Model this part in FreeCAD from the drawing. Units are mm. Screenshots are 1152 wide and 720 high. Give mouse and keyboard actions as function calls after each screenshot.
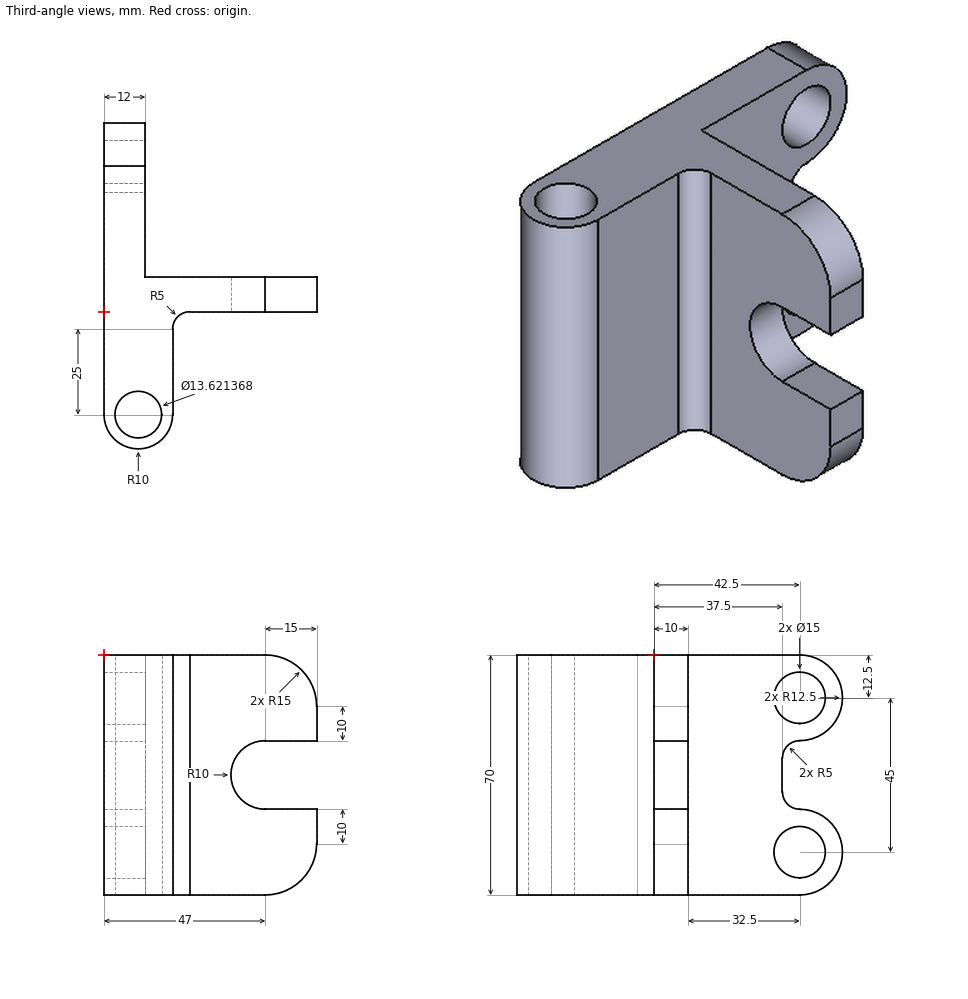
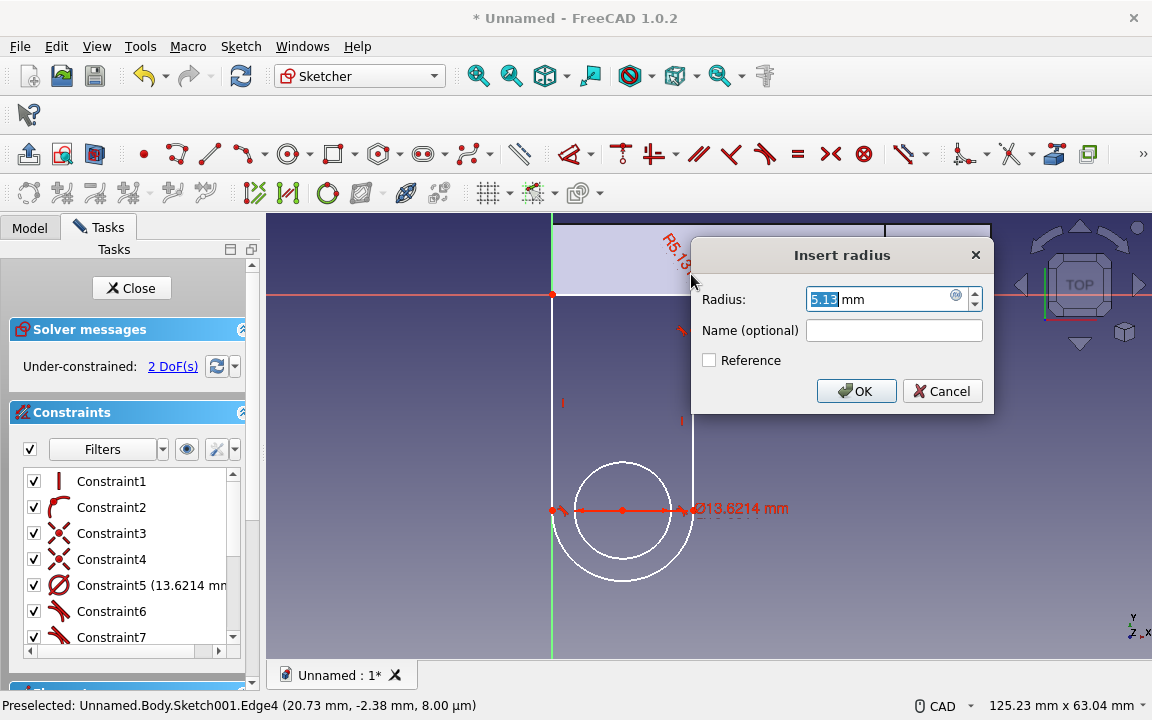
text(5)
key(Return)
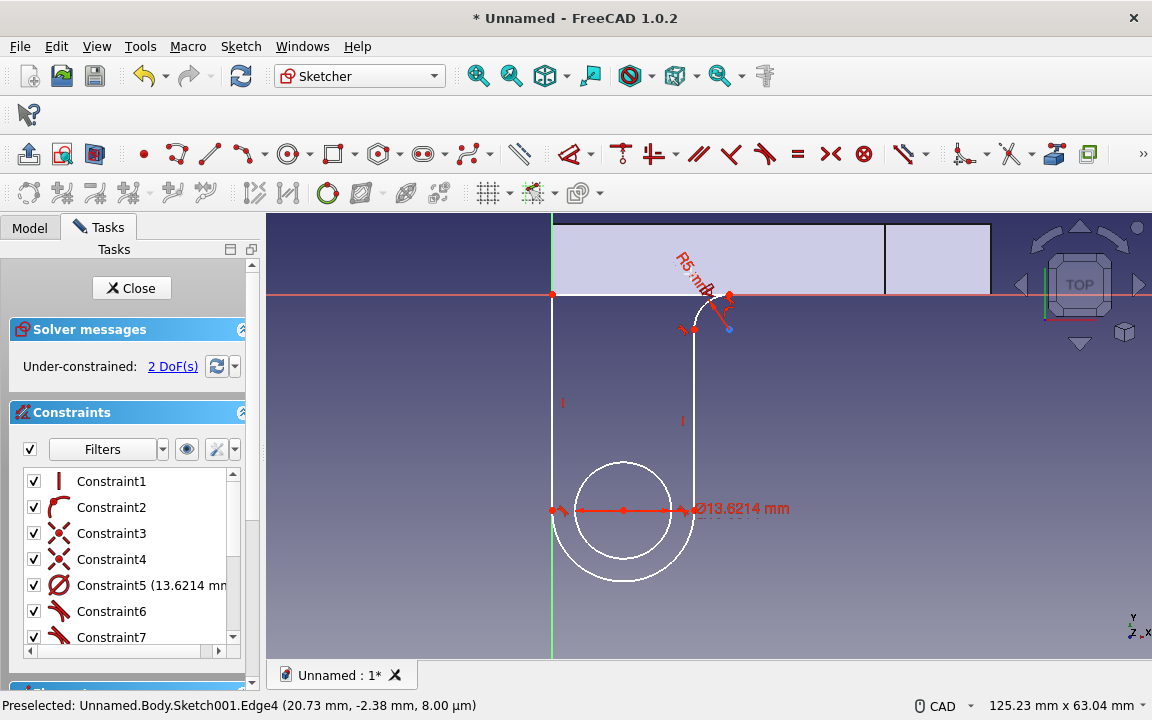
click(582, 568)
click(531, 555)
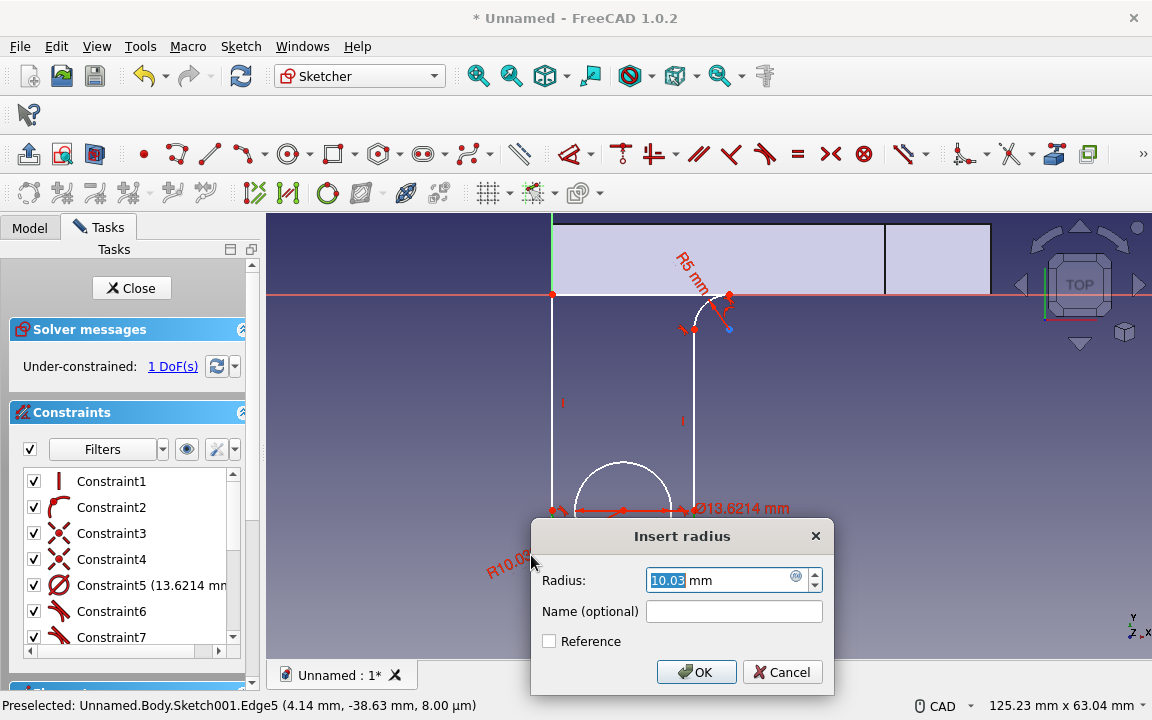
text(10)
key(Return)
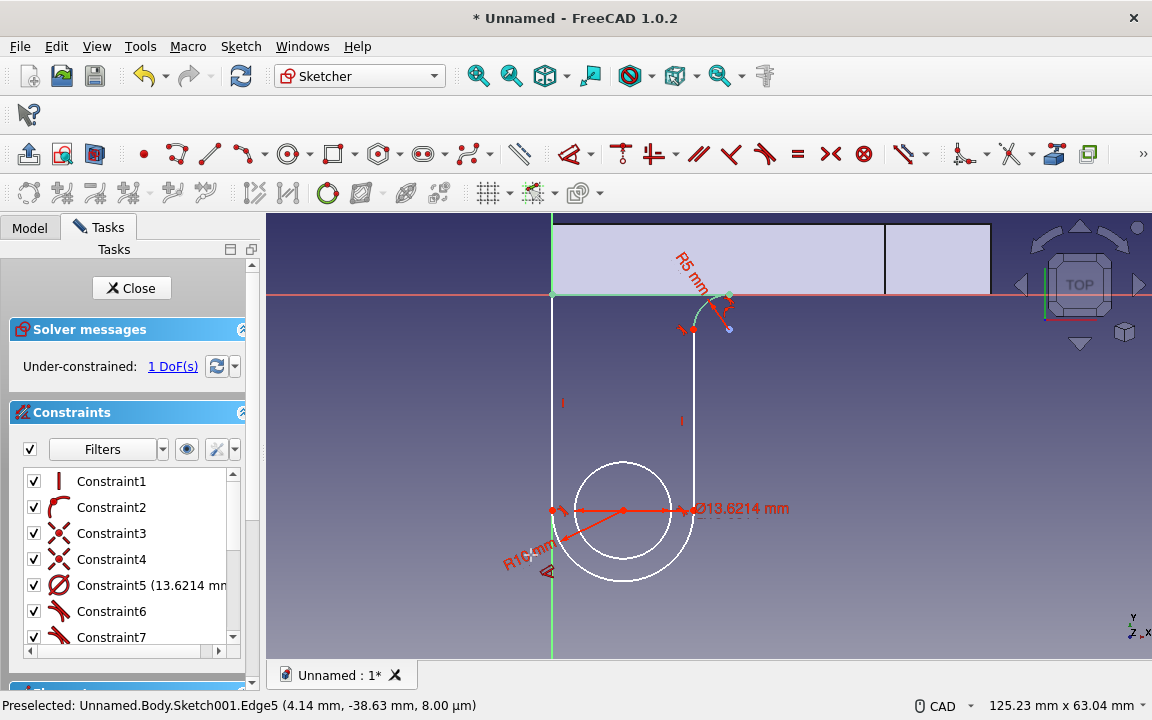
click(694, 456)
click(728, 420)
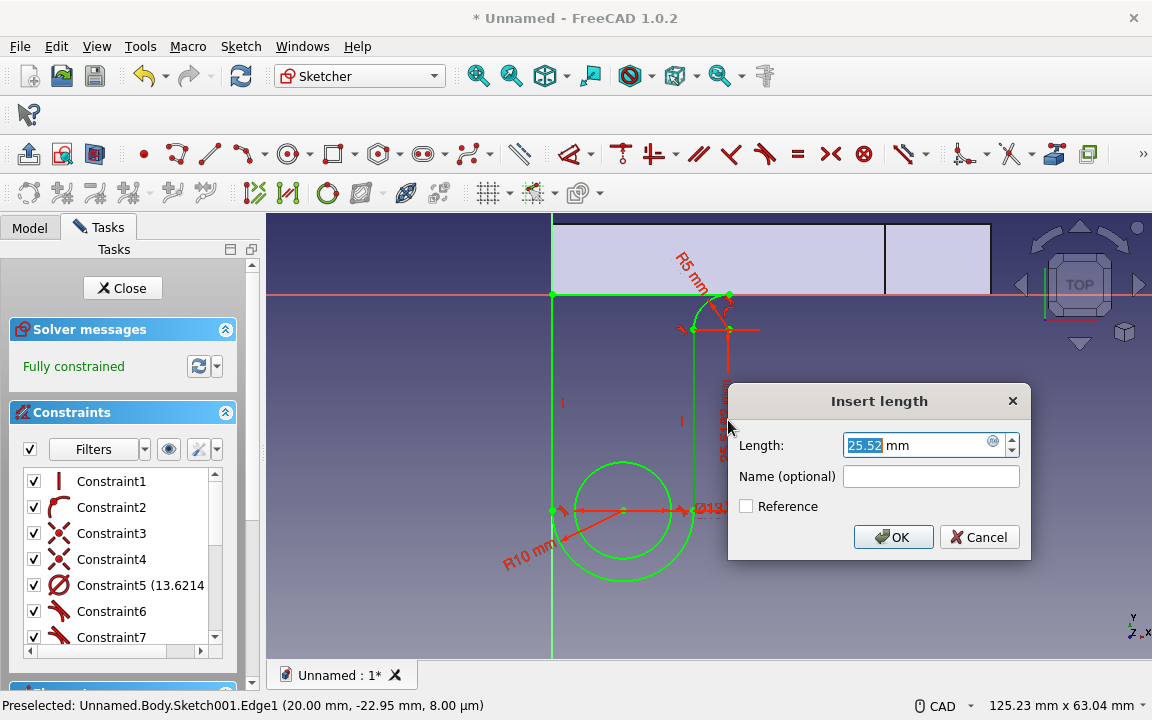
text(25)
key(Return)
key(Escape)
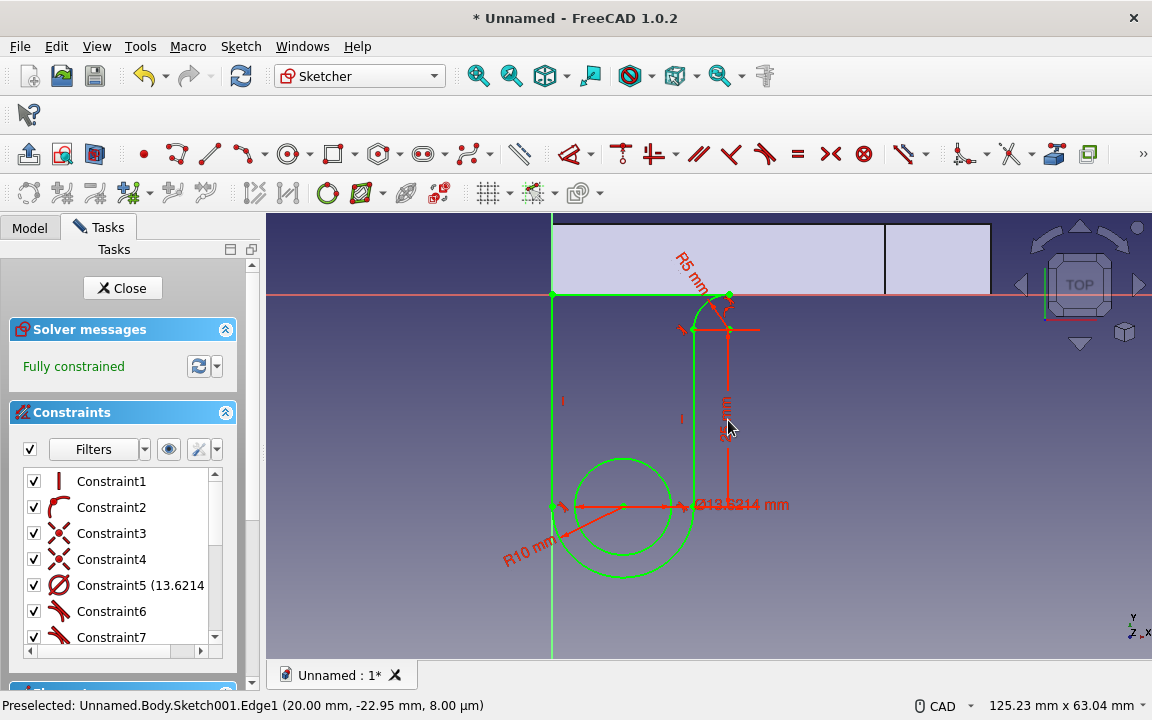
click(123, 288)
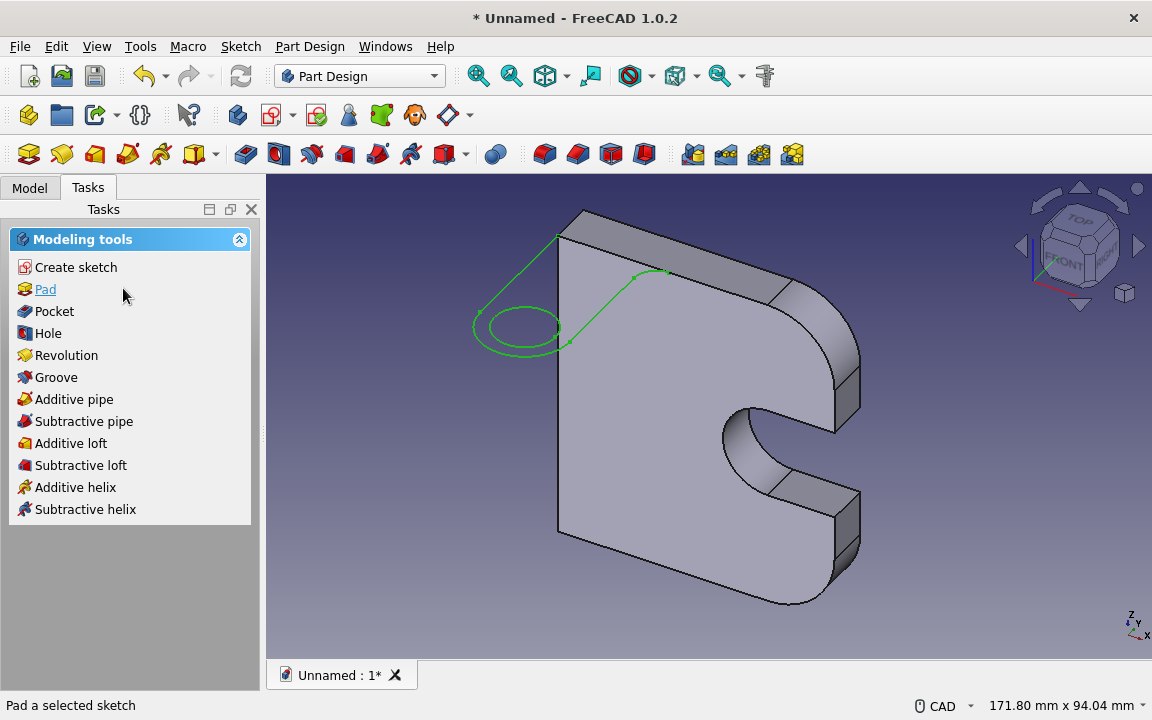
click(29, 154)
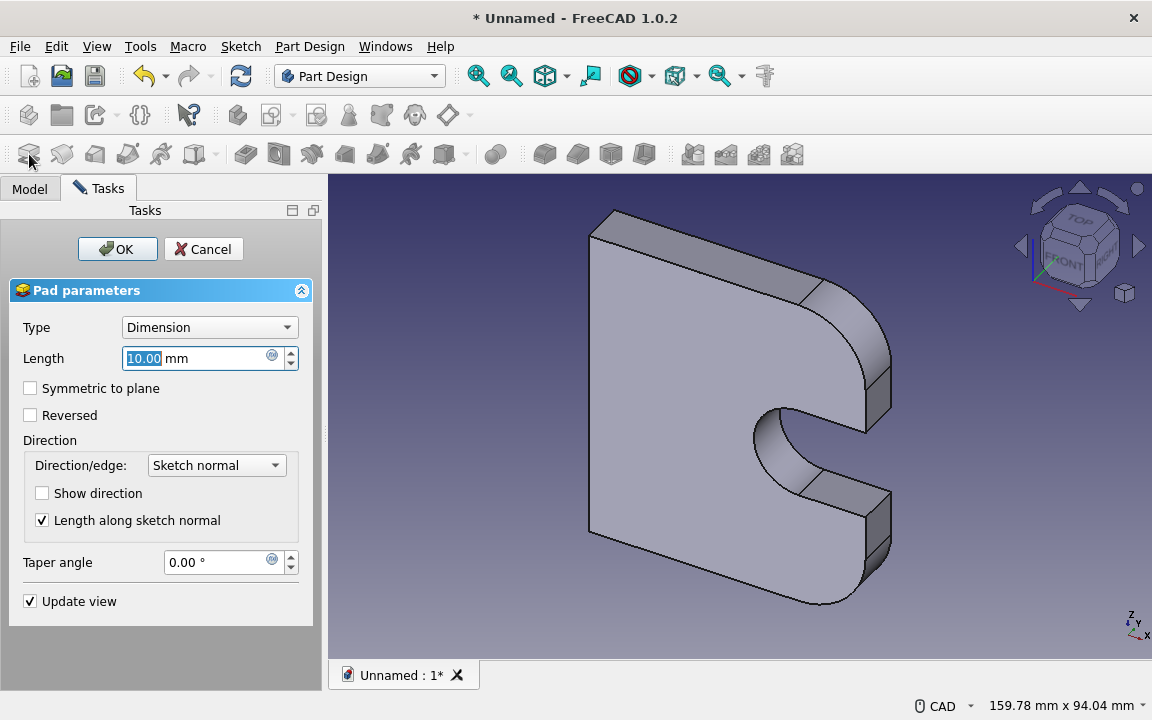
text(70)
key(Tab)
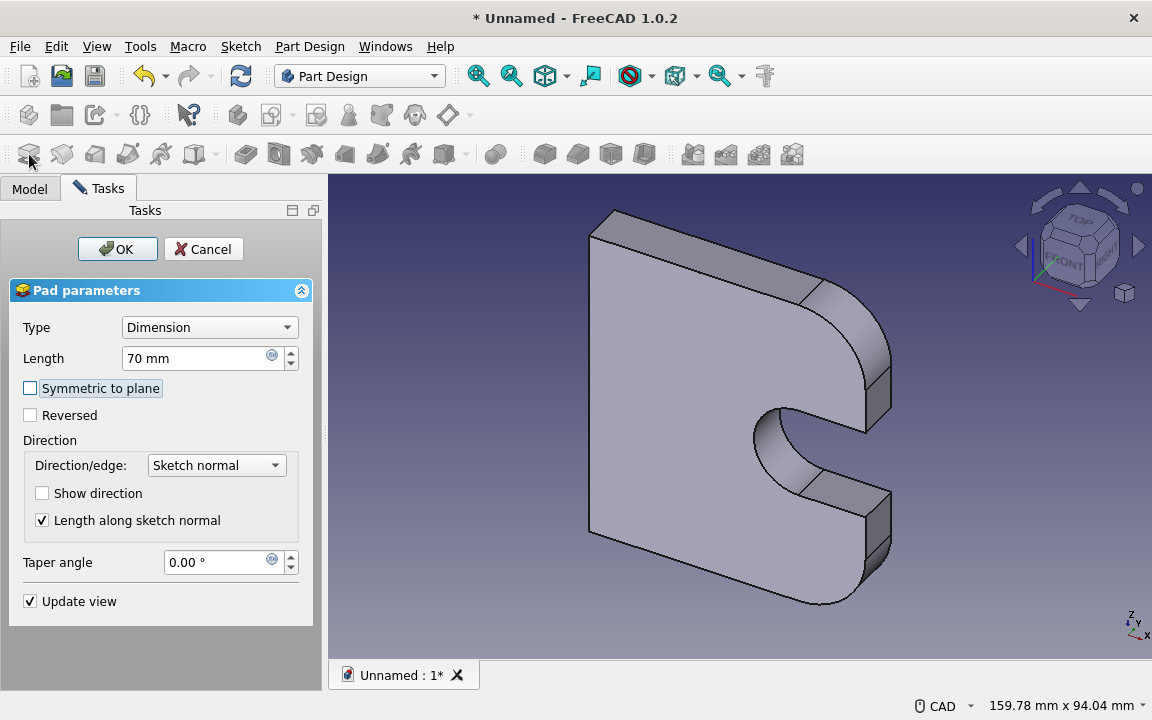
click(31, 415)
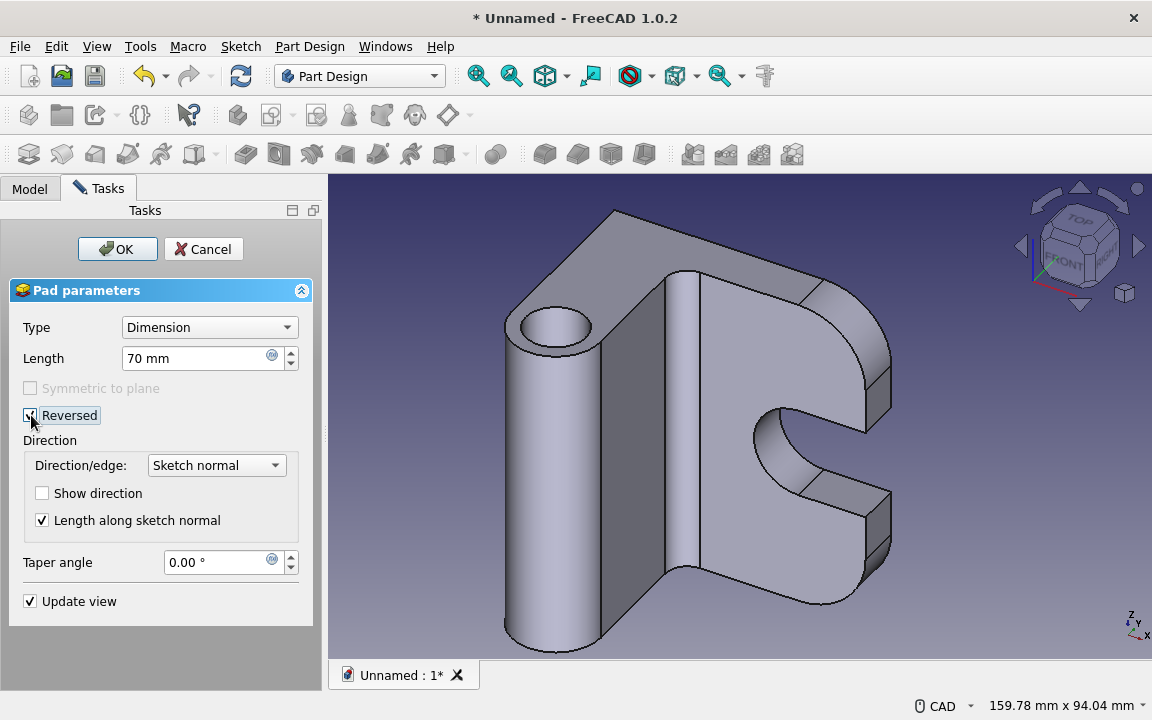
click(118, 249)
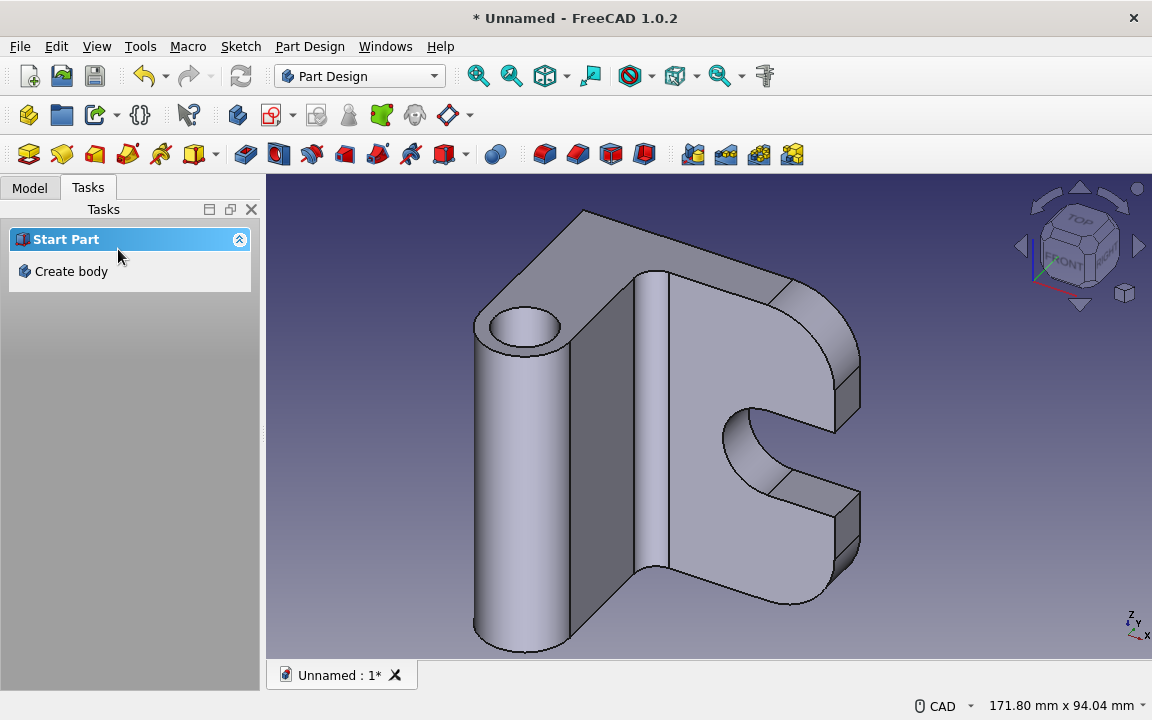
click(479, 76)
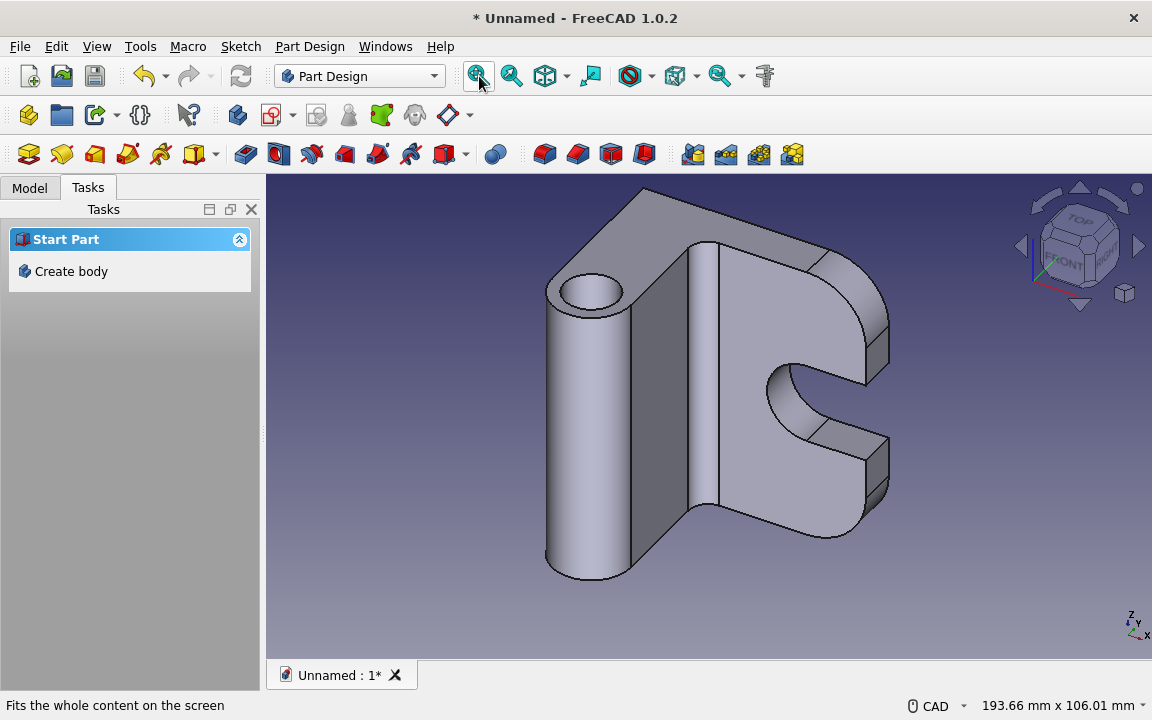
click(270, 116)